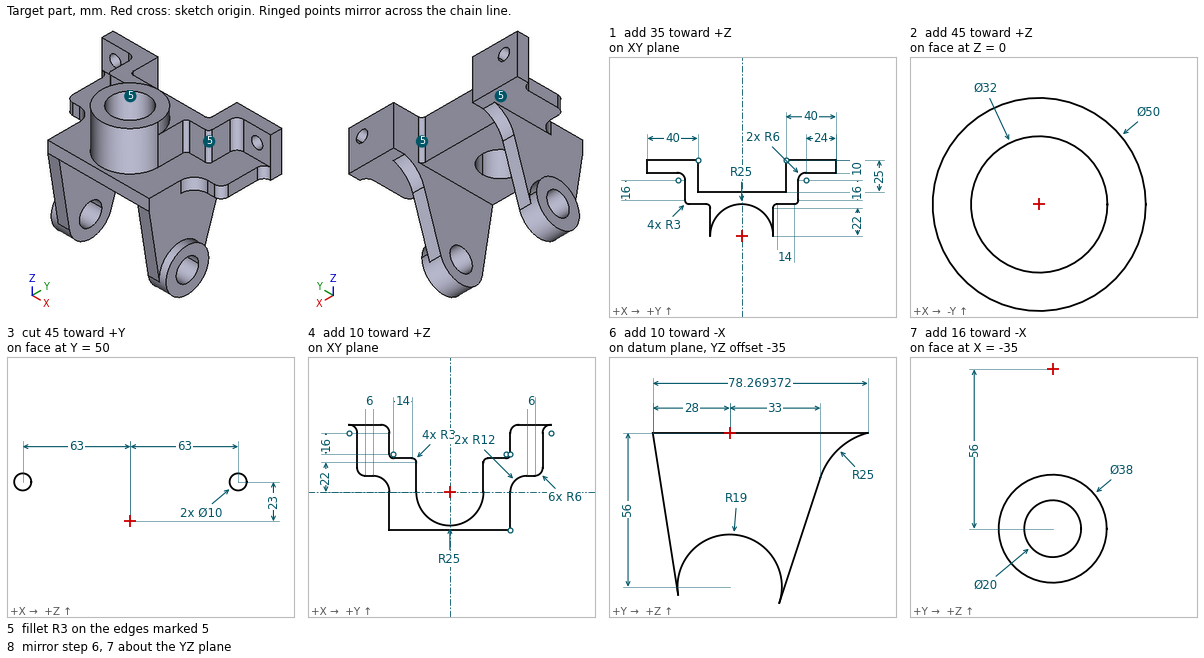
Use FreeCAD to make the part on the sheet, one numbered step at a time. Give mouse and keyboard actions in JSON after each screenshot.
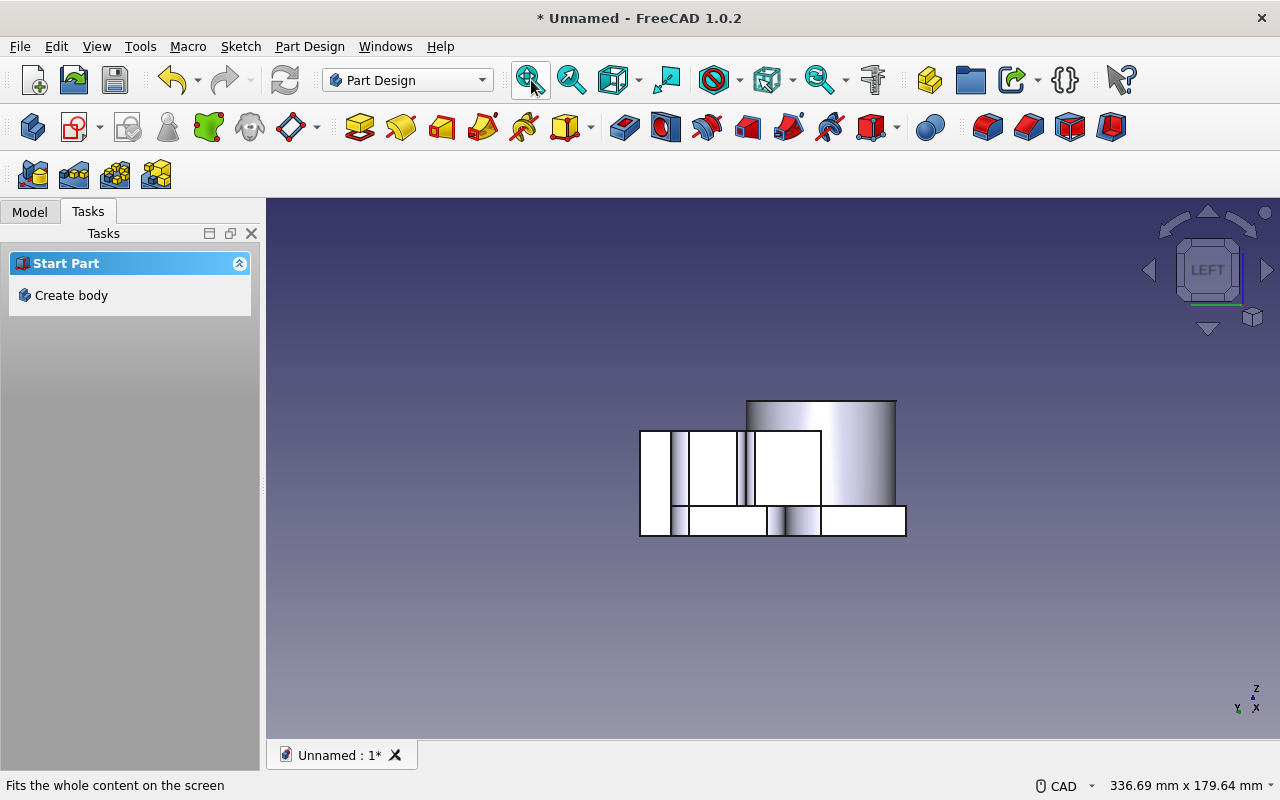
{"action": "key", "text": "v 3"}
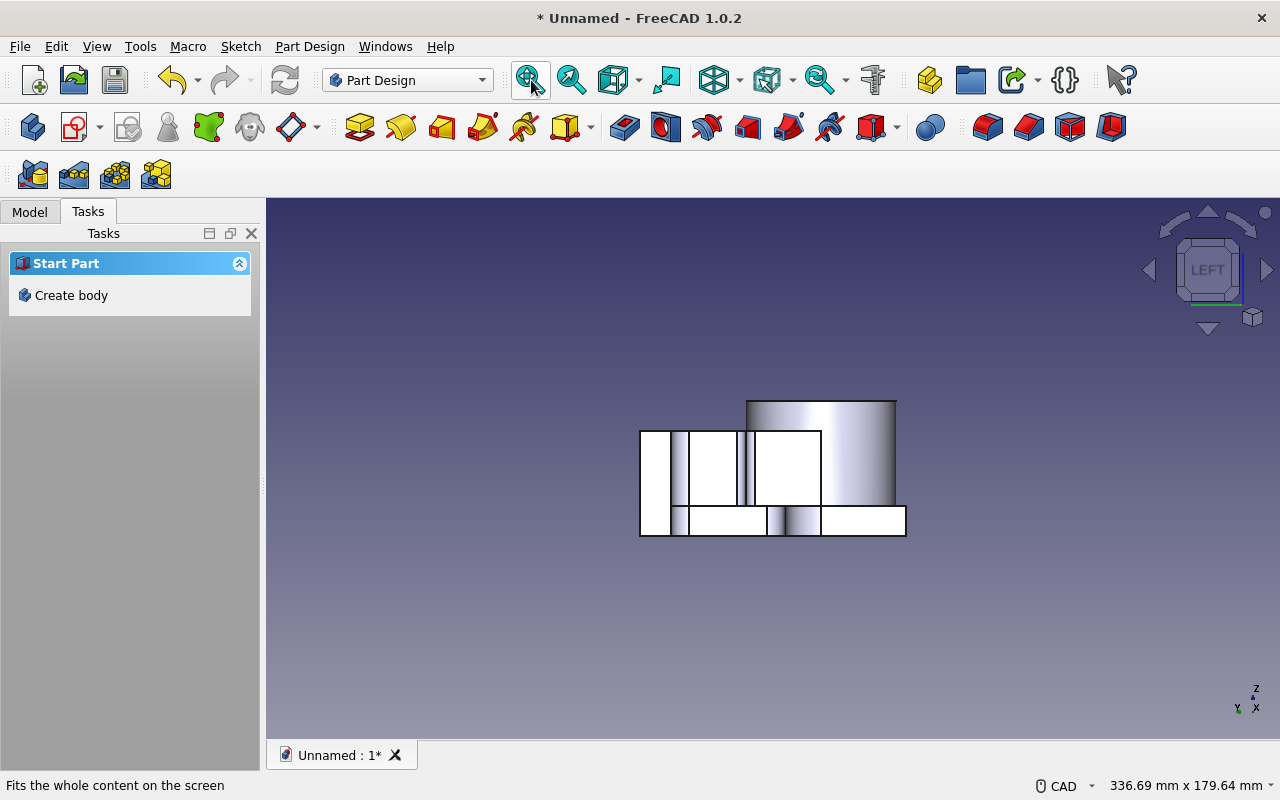
{"action": "key", "text": "0"}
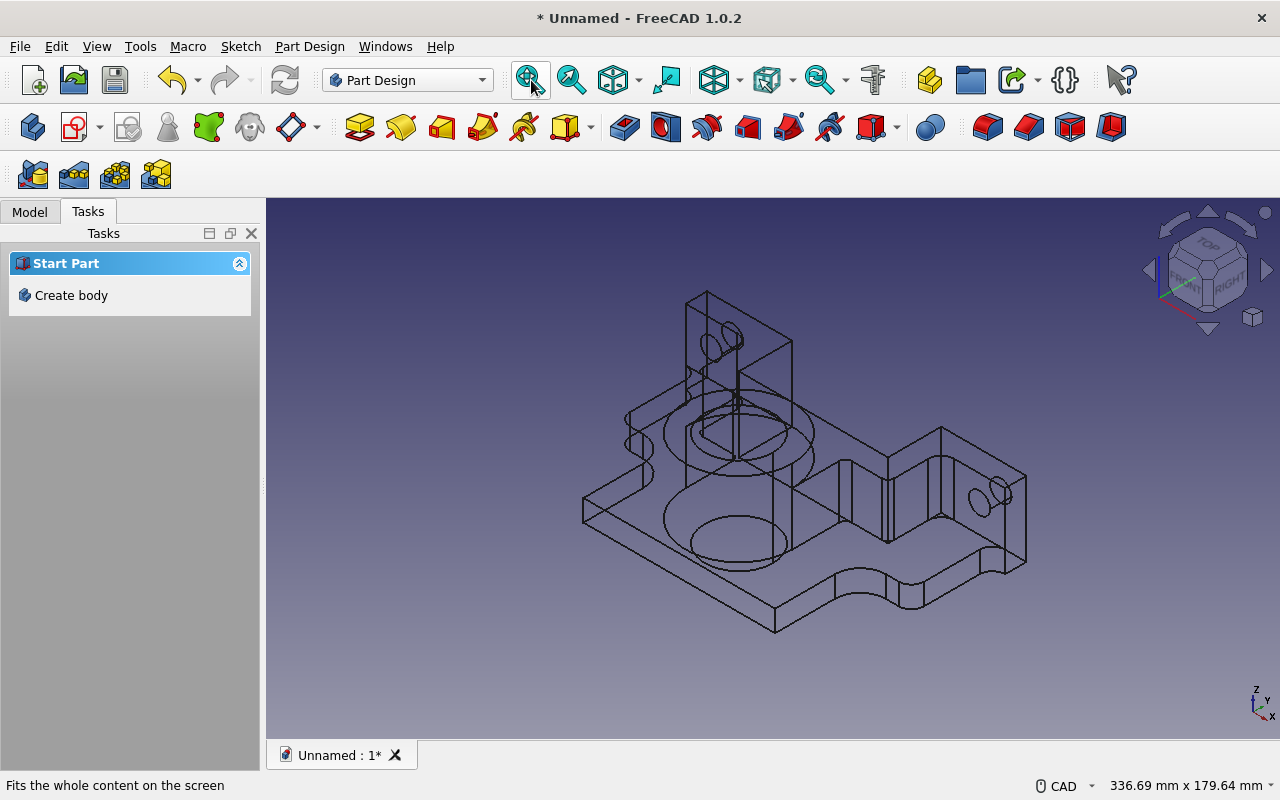
{"action": "left_click", "coordinate": [888, 499]}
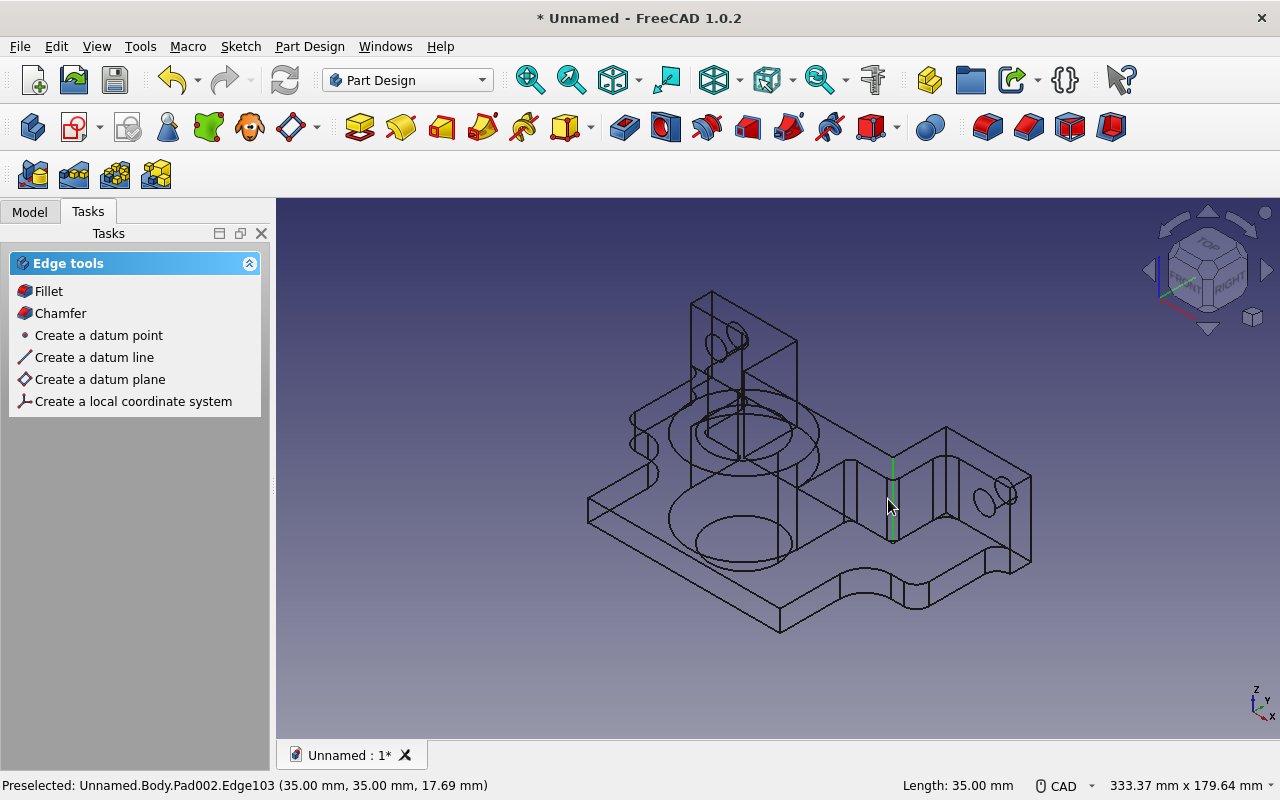
{"action": "left_click", "coordinate": [744, 422], "text": "ctrl"}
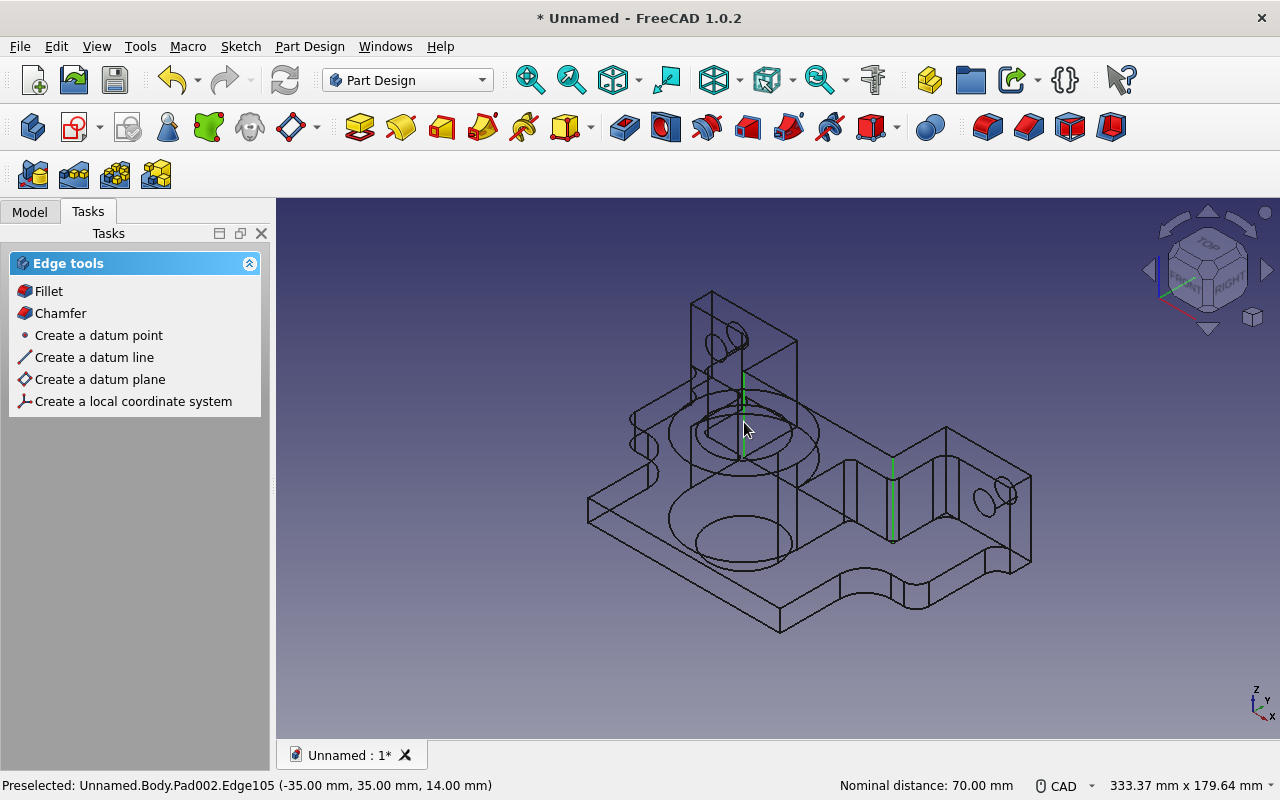
{"action": "key", "text": "v 1"}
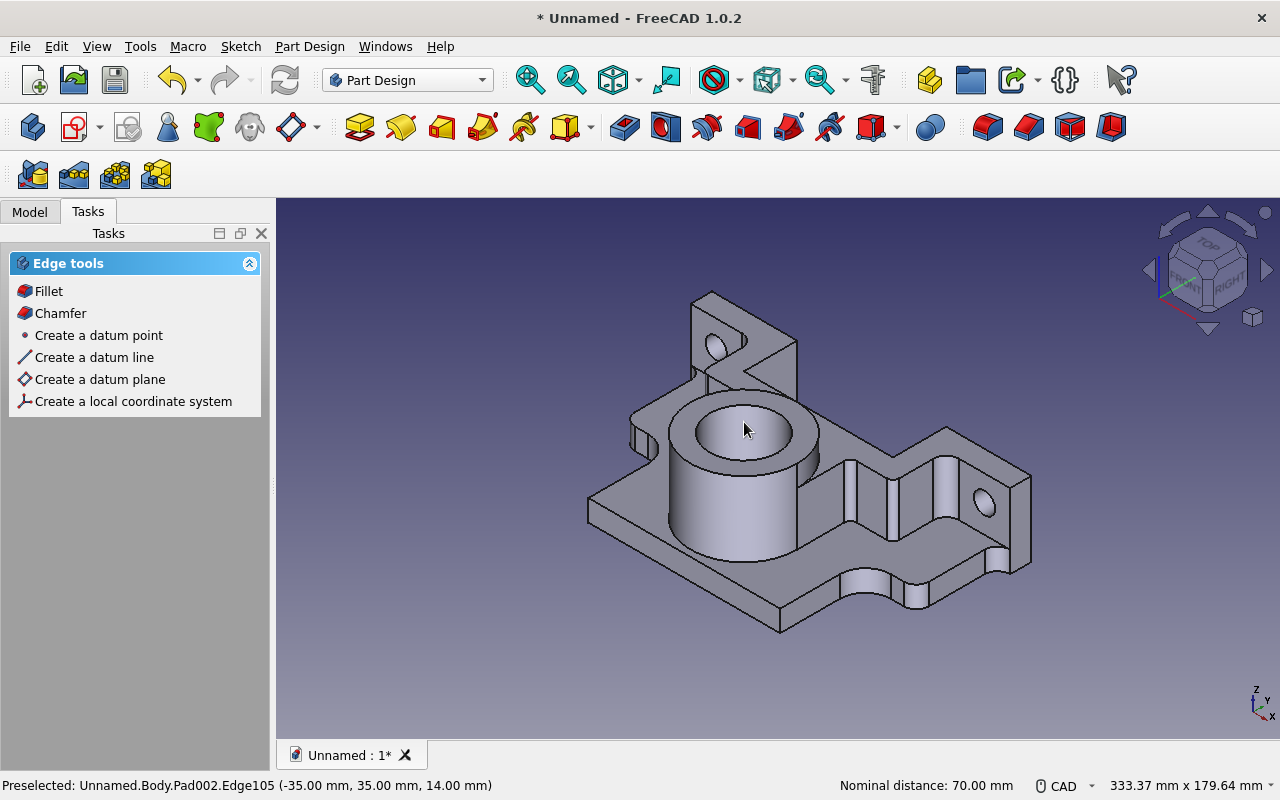
{"action": "left_click", "coordinate": [988, 128]}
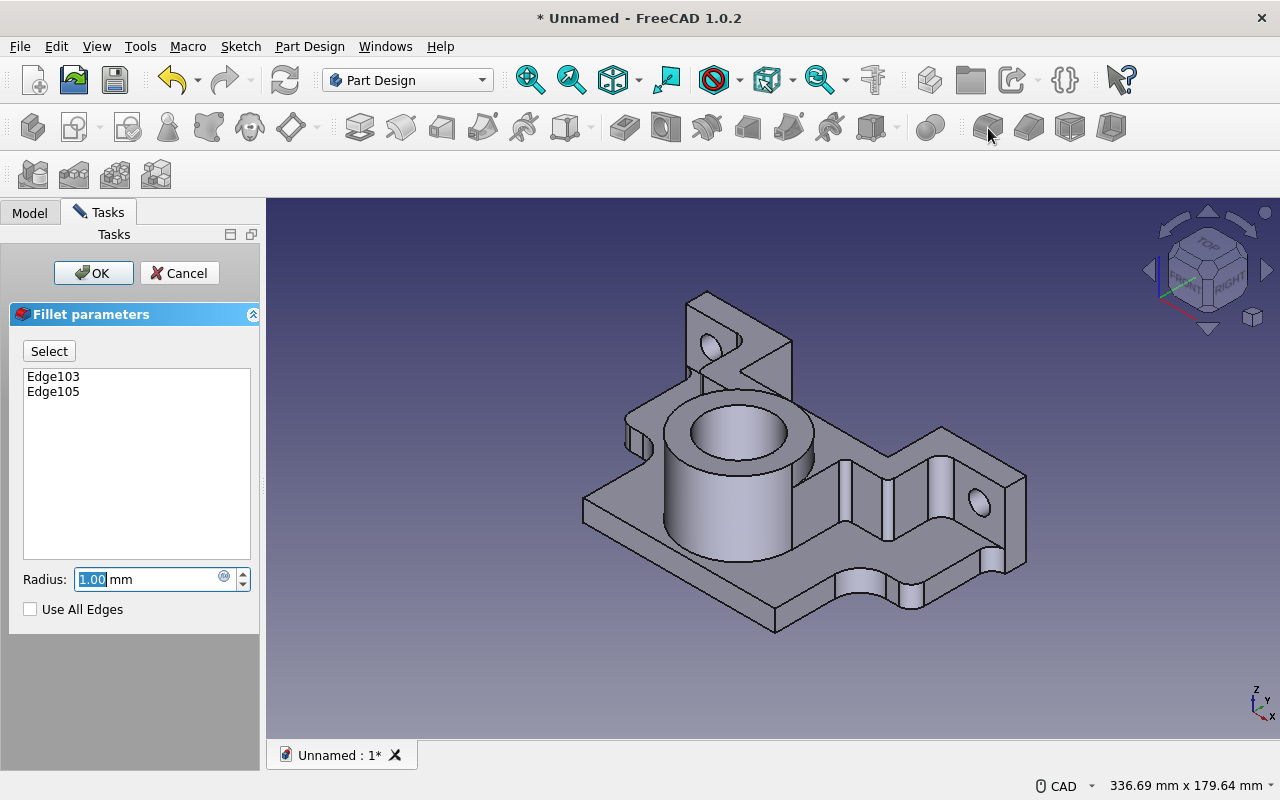
{"action": "type", "text": "3"}
{"action": "key", "text": "Tab"}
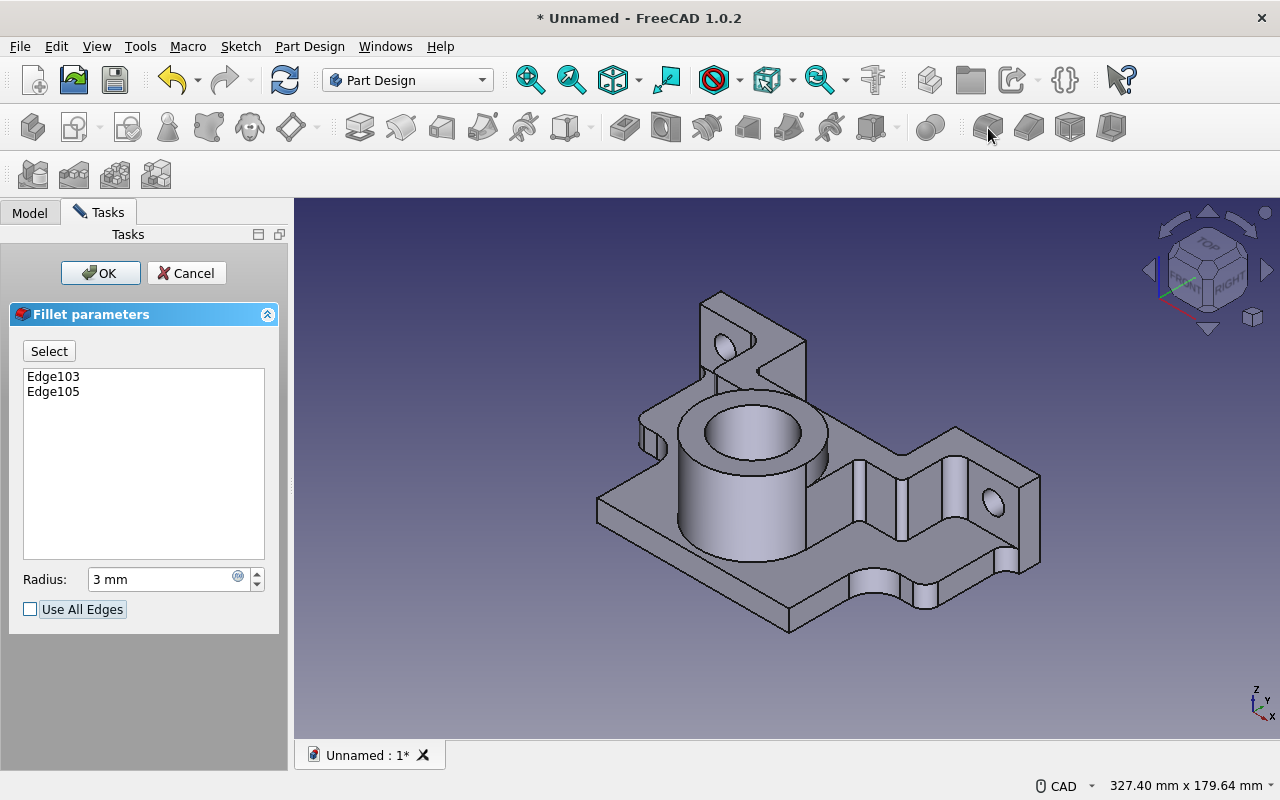
{"action": "left_click", "coordinate": [101, 273]}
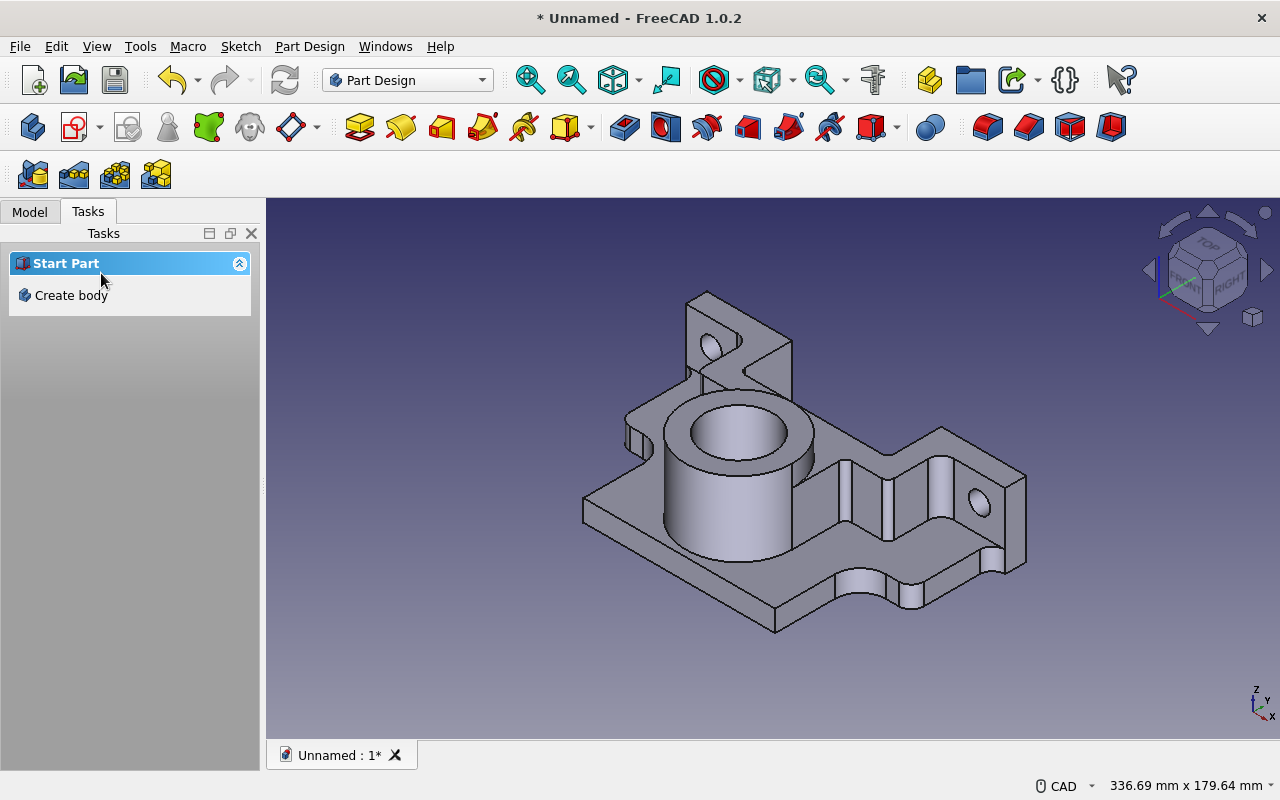
{"action": "left_click", "coordinate": [30, 212]}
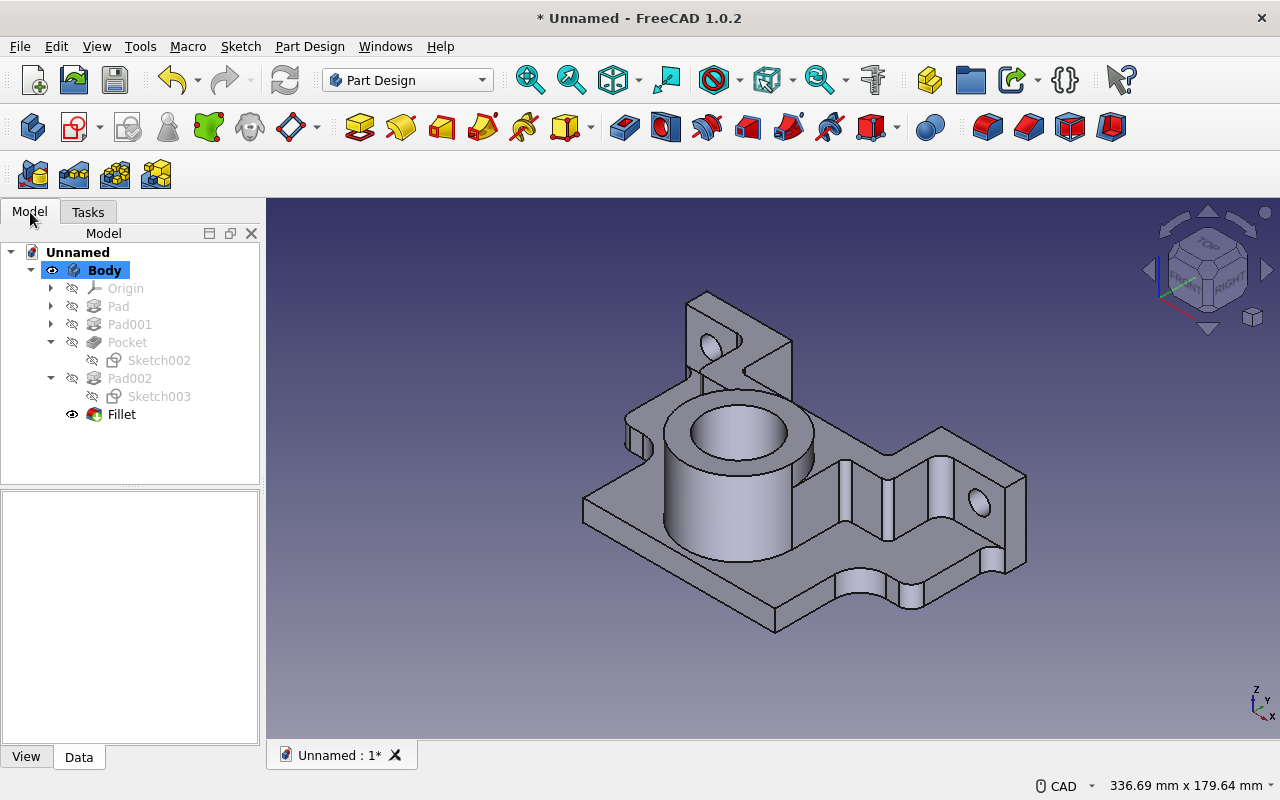
{"action": "left_click", "coordinate": [51, 288]}